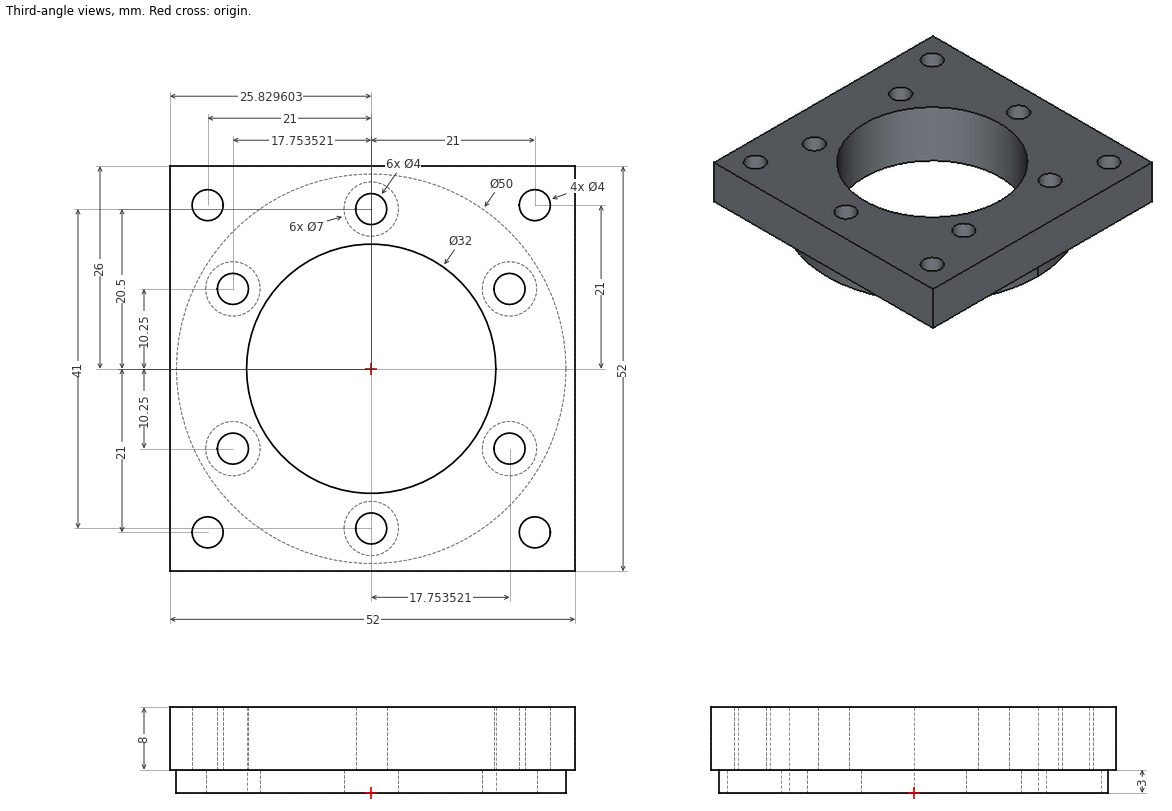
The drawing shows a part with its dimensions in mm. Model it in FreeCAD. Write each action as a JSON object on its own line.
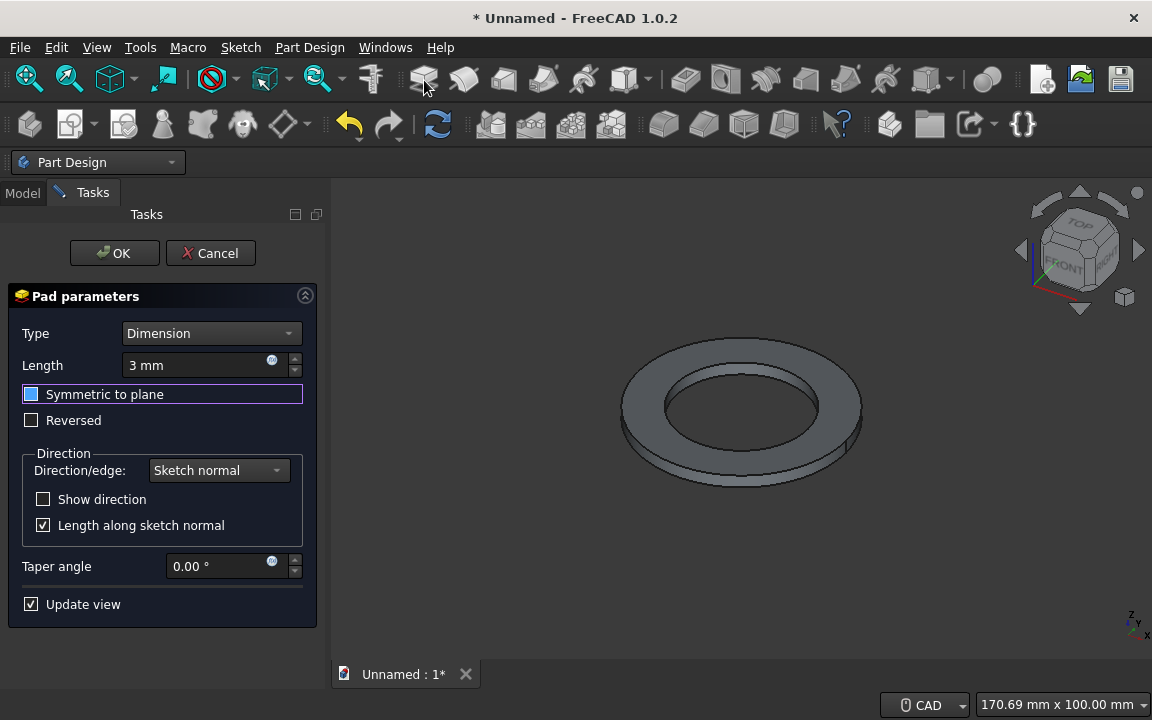
{"action": "left_click", "coordinate": [115, 253]}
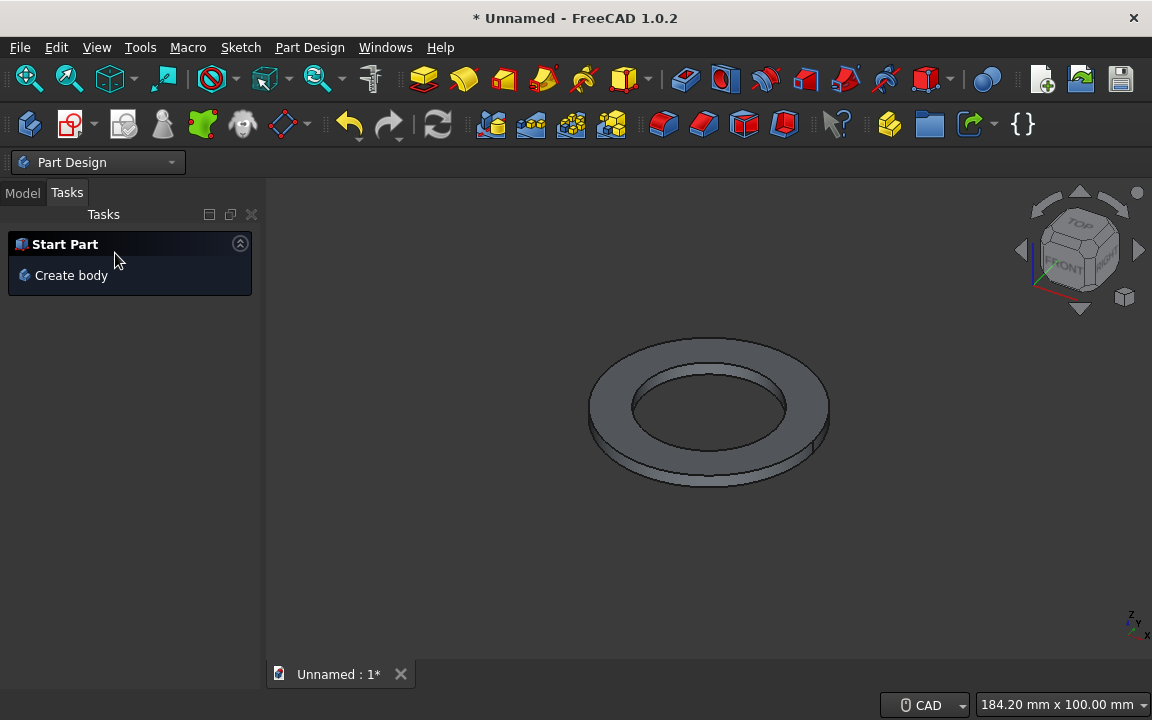
{"action": "key", "text": "v f"}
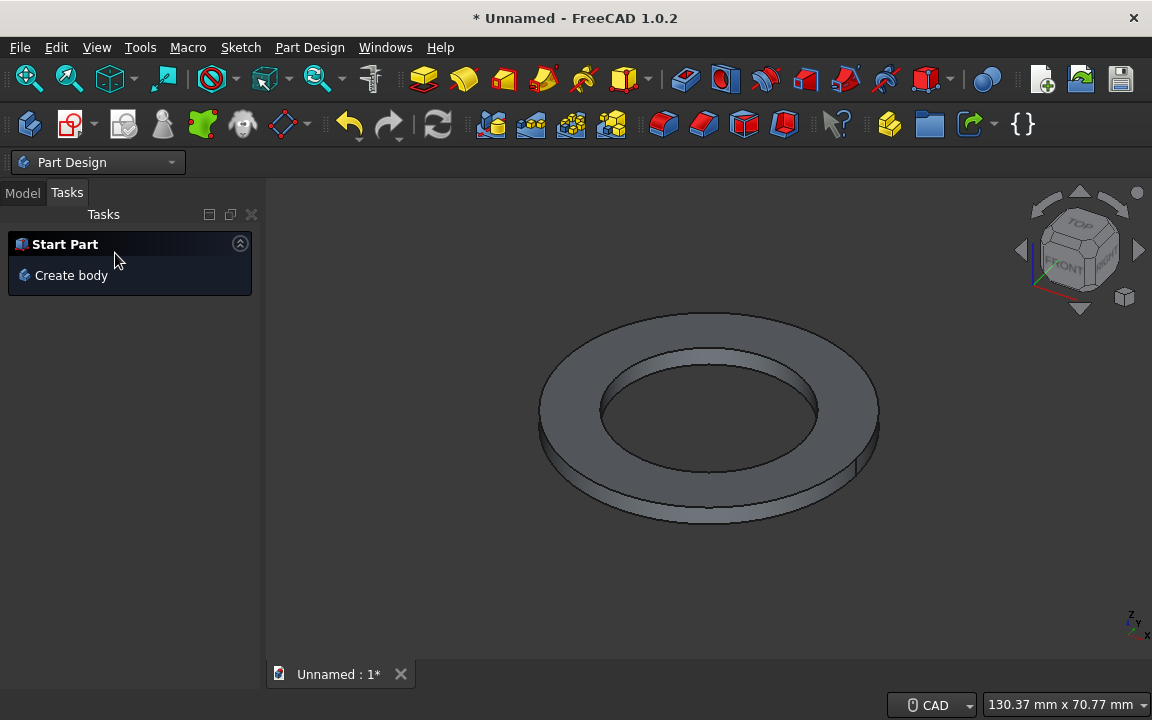
{"action": "left_click", "coordinate": [673, 333]}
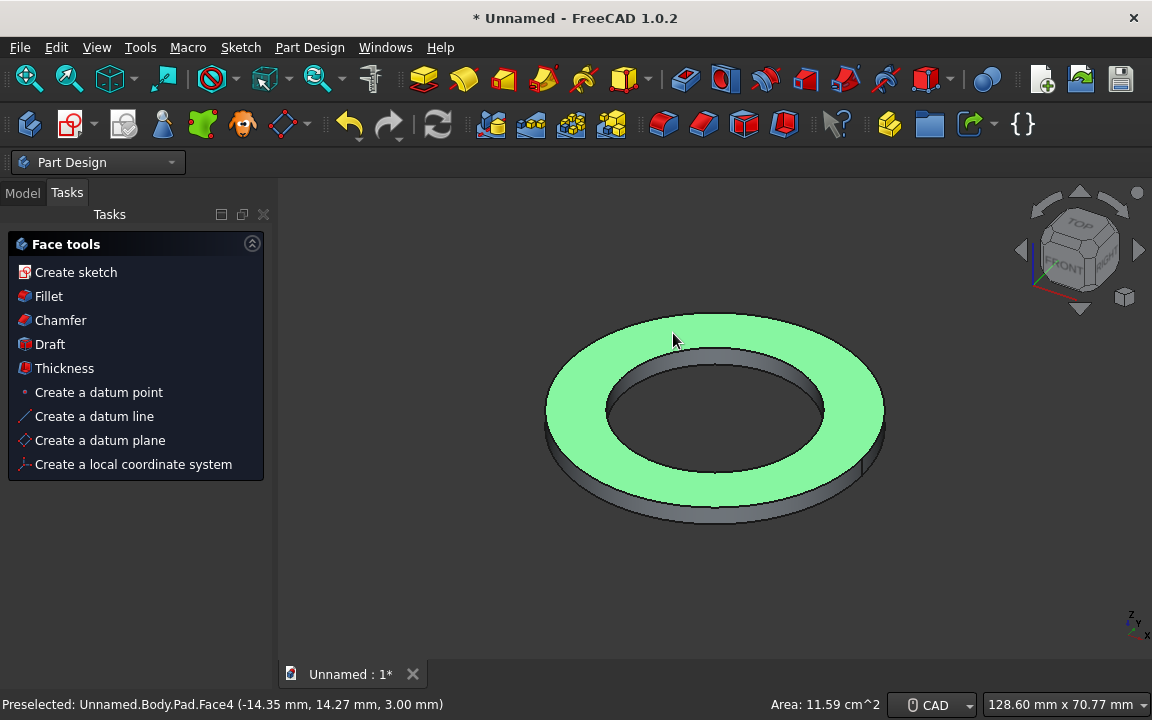
{"action": "left_click", "coordinate": [70, 124]}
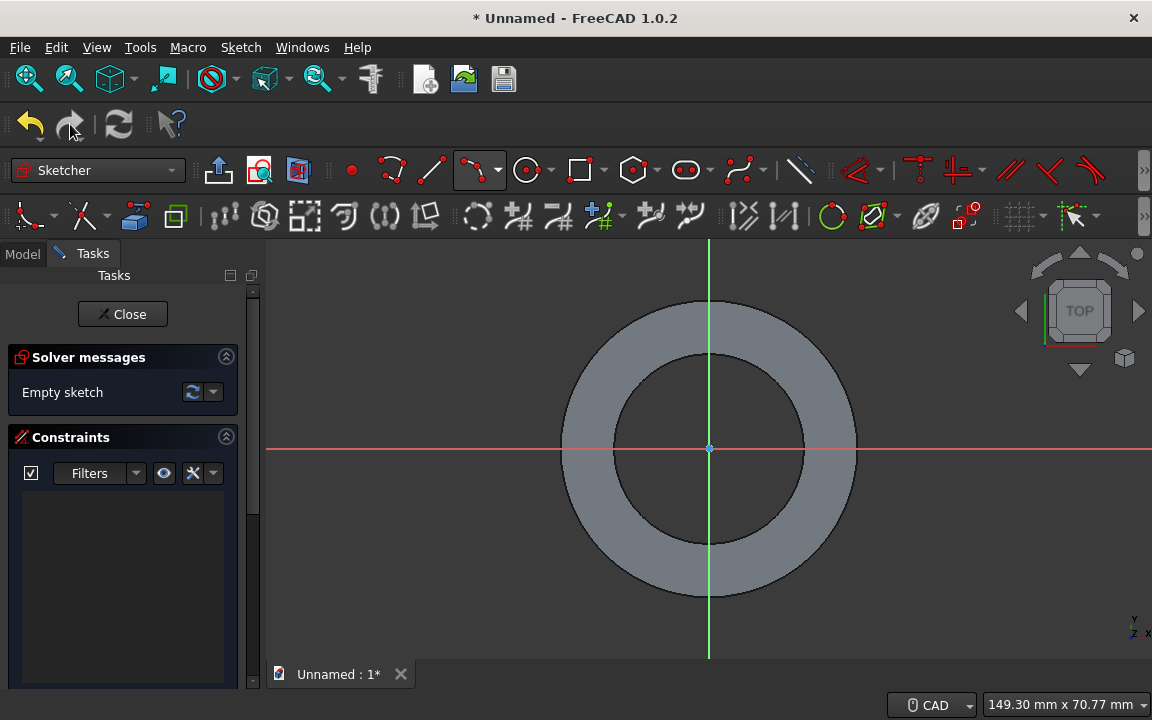
{"action": "key", "text": "g r"}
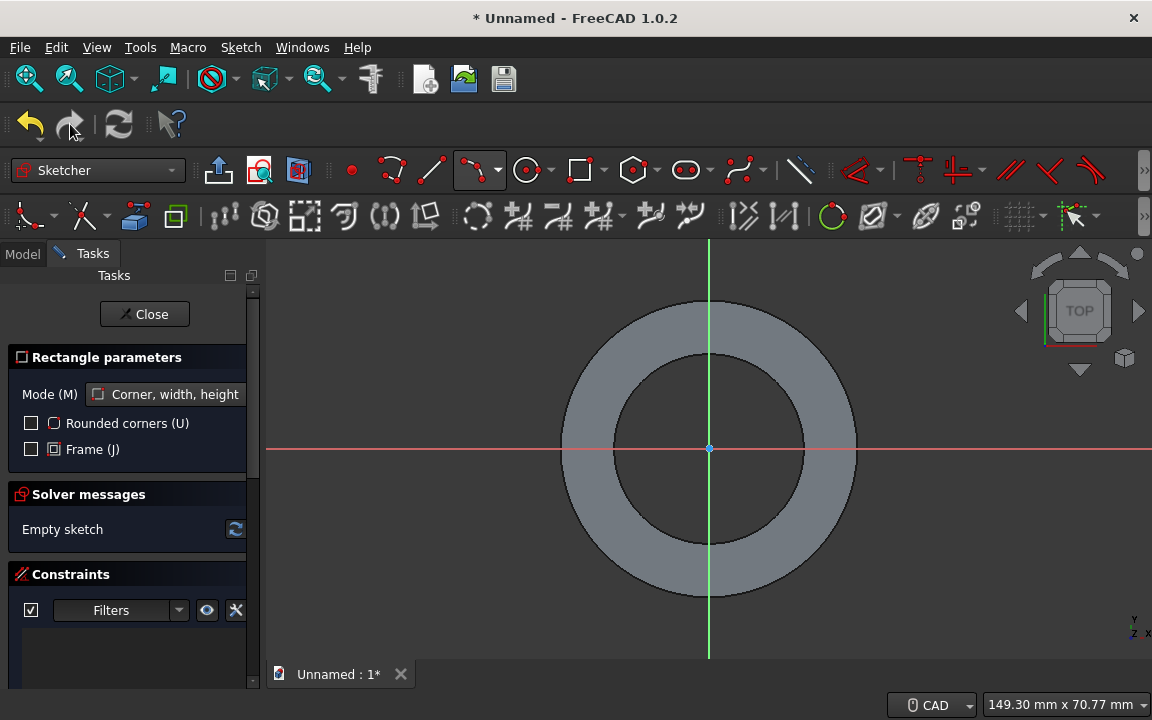
{"action": "left_click", "coordinate": [556, 295]}
{"action": "mouse_move", "coordinate": [864, 603]}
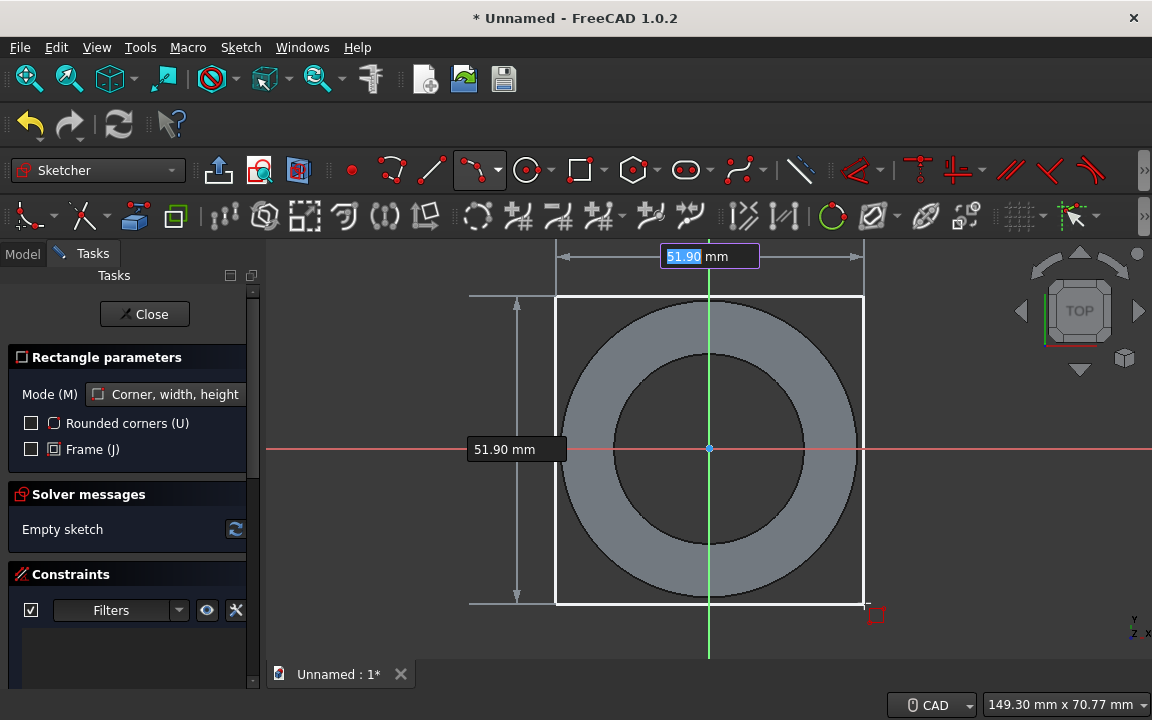
{"action": "type", "text": "52"}
{"action": "key", "text": "Tab"}
{"action": "type", "text": "52"}
{"action": "key", "text": "Return"}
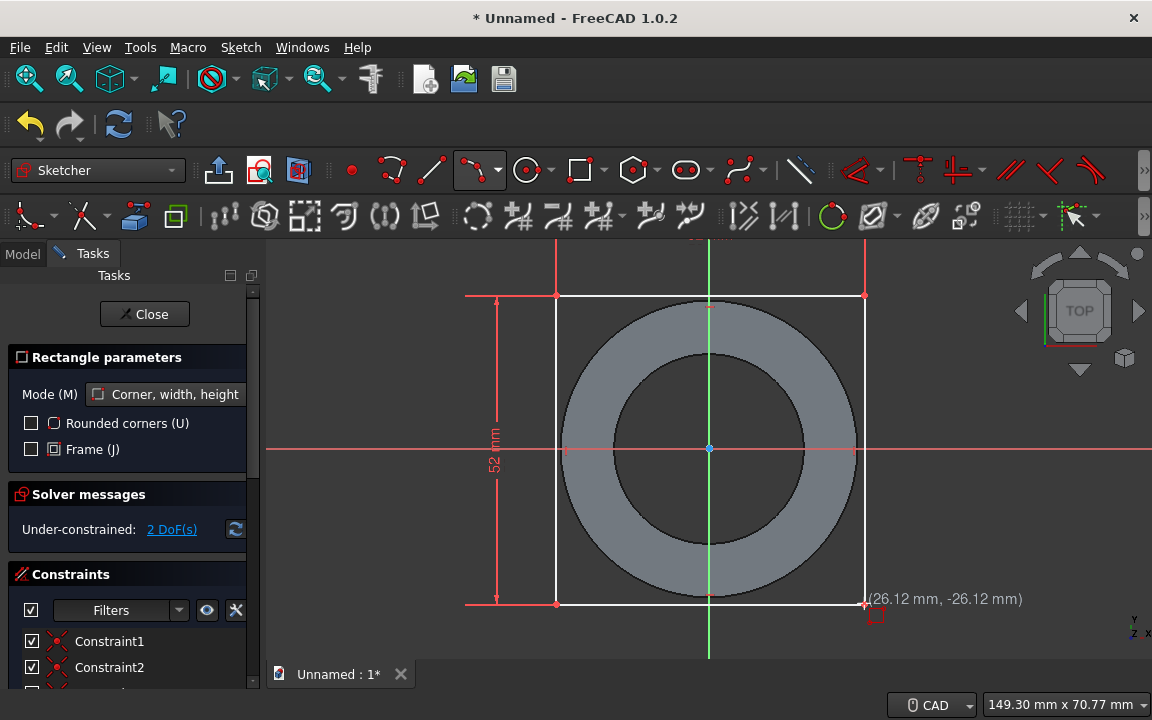
{"action": "key", "text": "g c"}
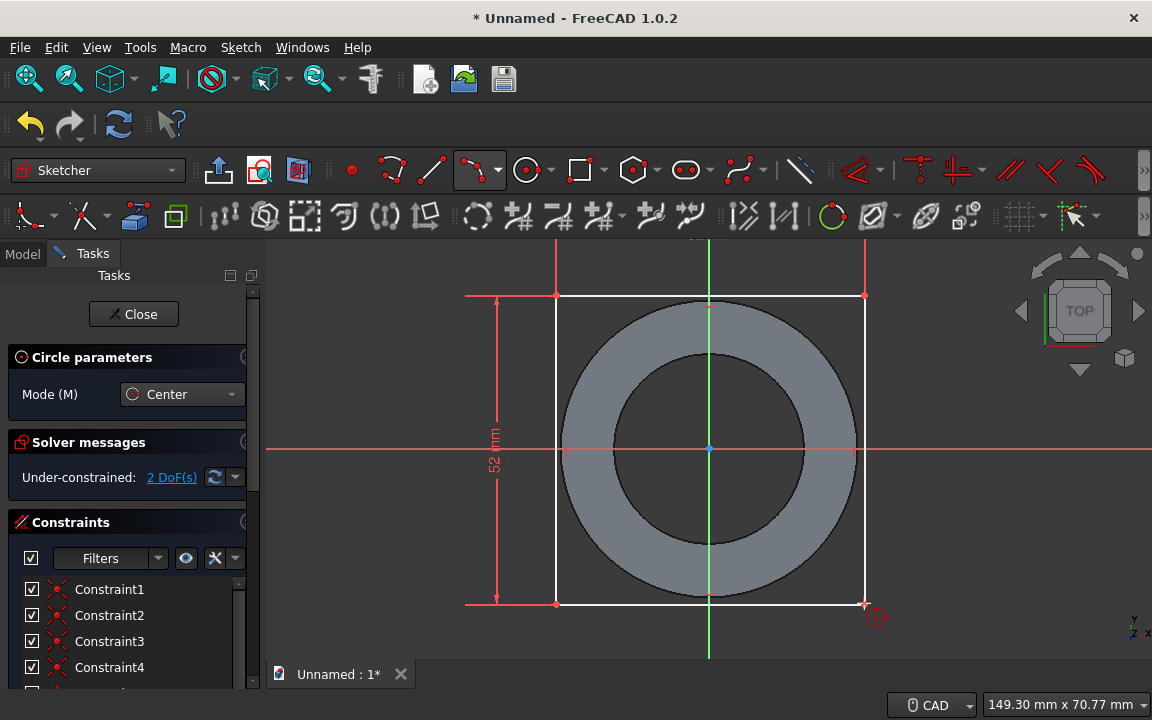
{"action": "left_click", "coordinate": [709, 449]}
{"action": "mouse_move", "coordinate": [776, 382]}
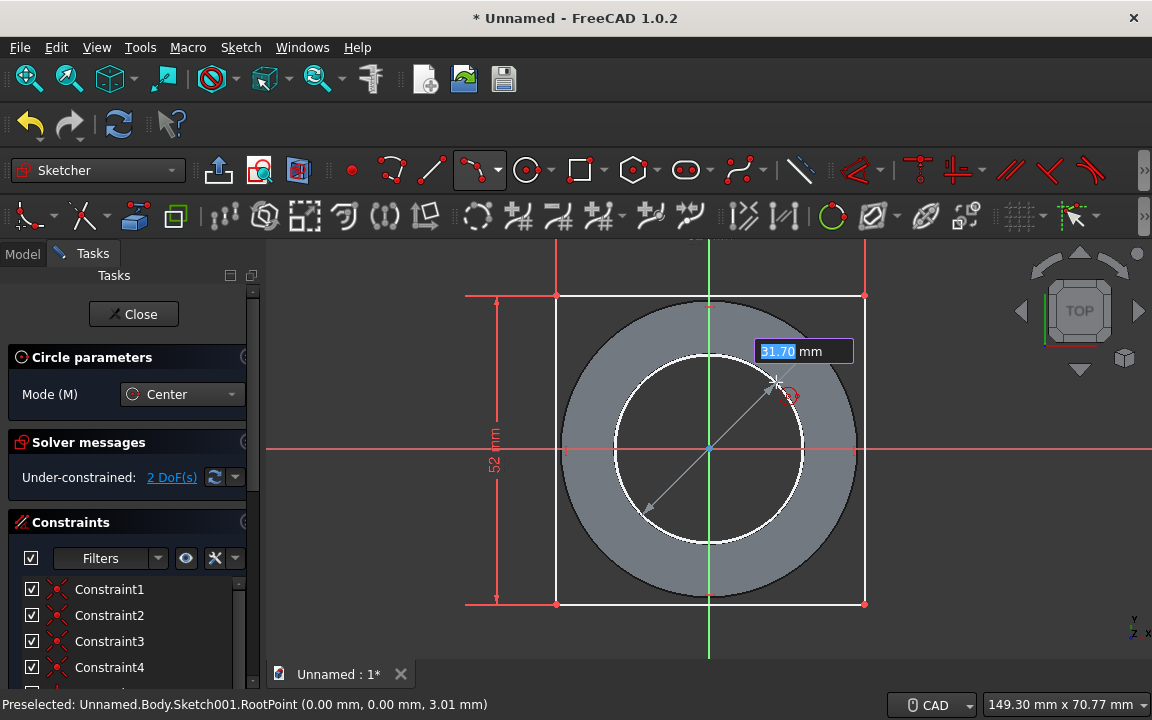
{"action": "type", "text": "32"}
{"action": "key", "text": "Return"}
{"action": "key", "text": "Escape"}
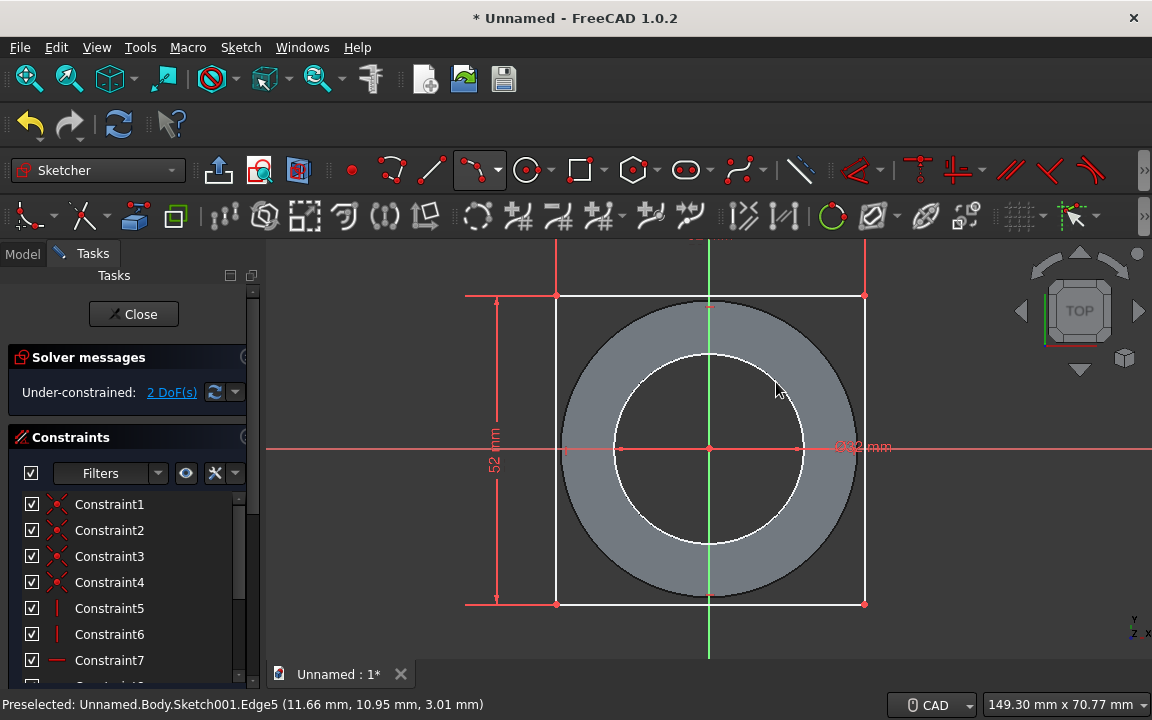
{"action": "key", "text": "d"}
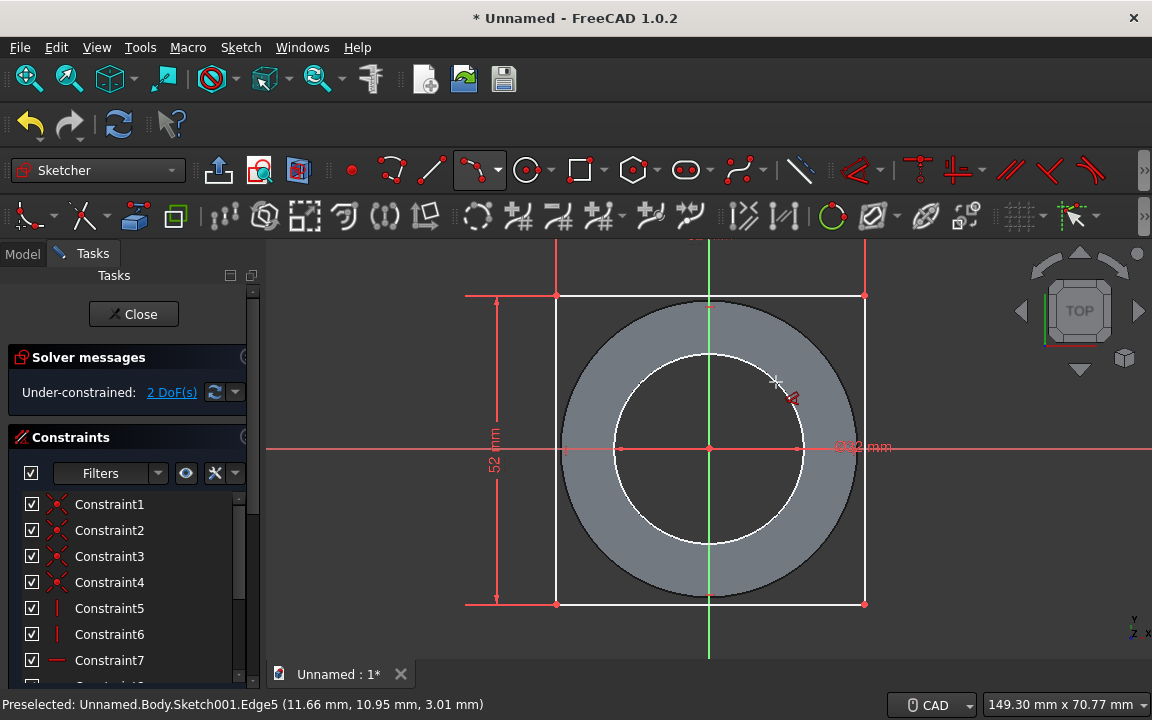
{"action": "left_click", "coordinate": [556, 296]}
{"action": "left_click", "coordinate": [522, 373]}